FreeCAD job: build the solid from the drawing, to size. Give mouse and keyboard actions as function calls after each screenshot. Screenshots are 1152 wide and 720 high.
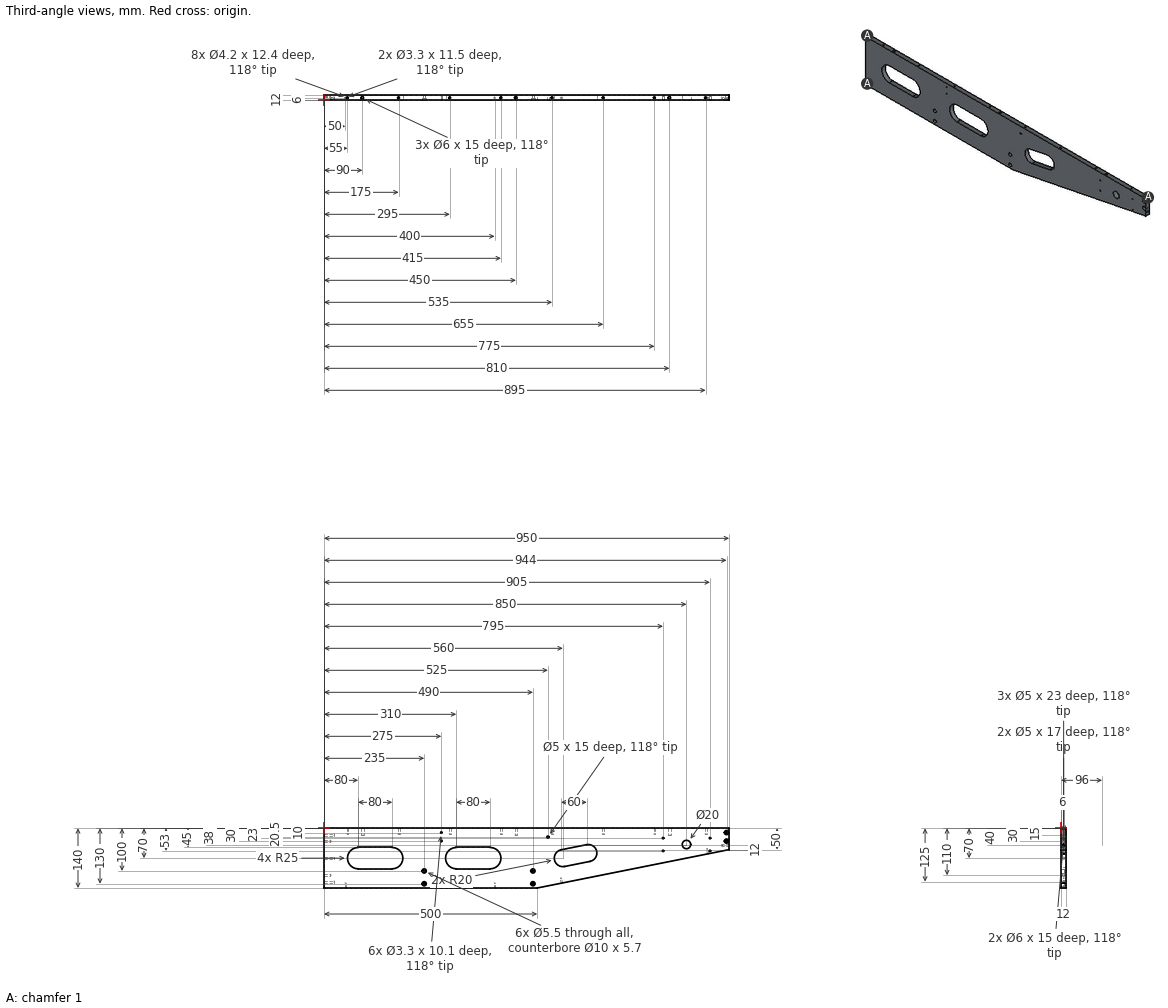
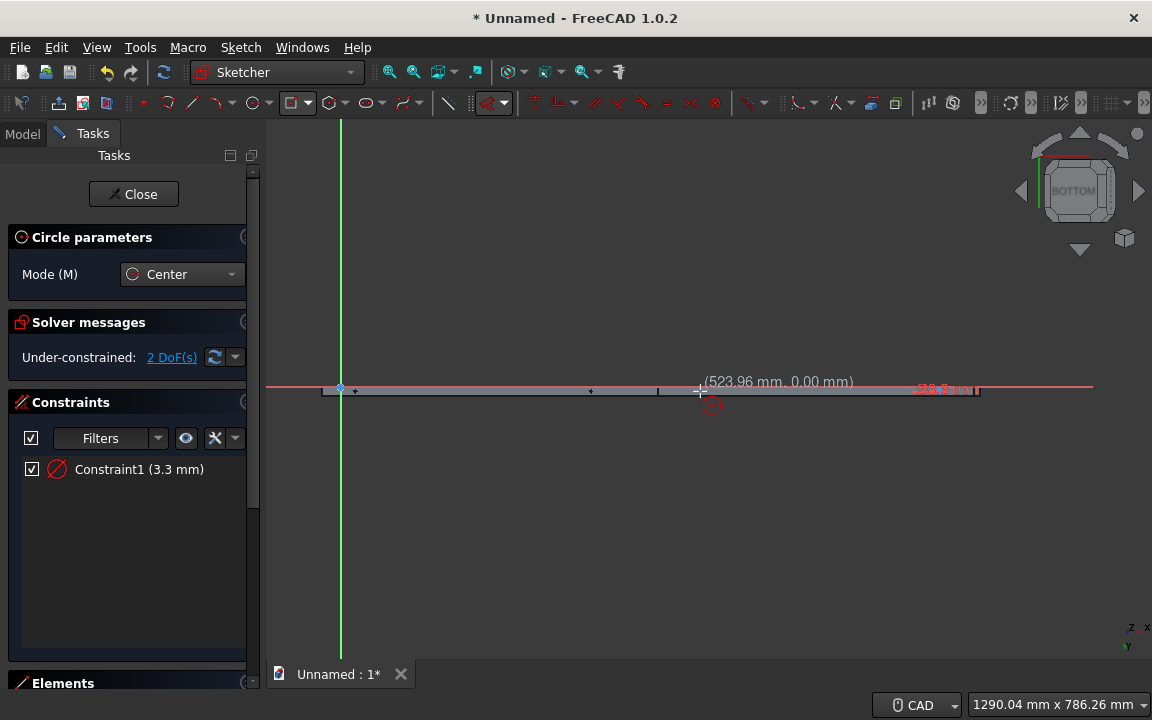
scroll(699, 391, up, 7)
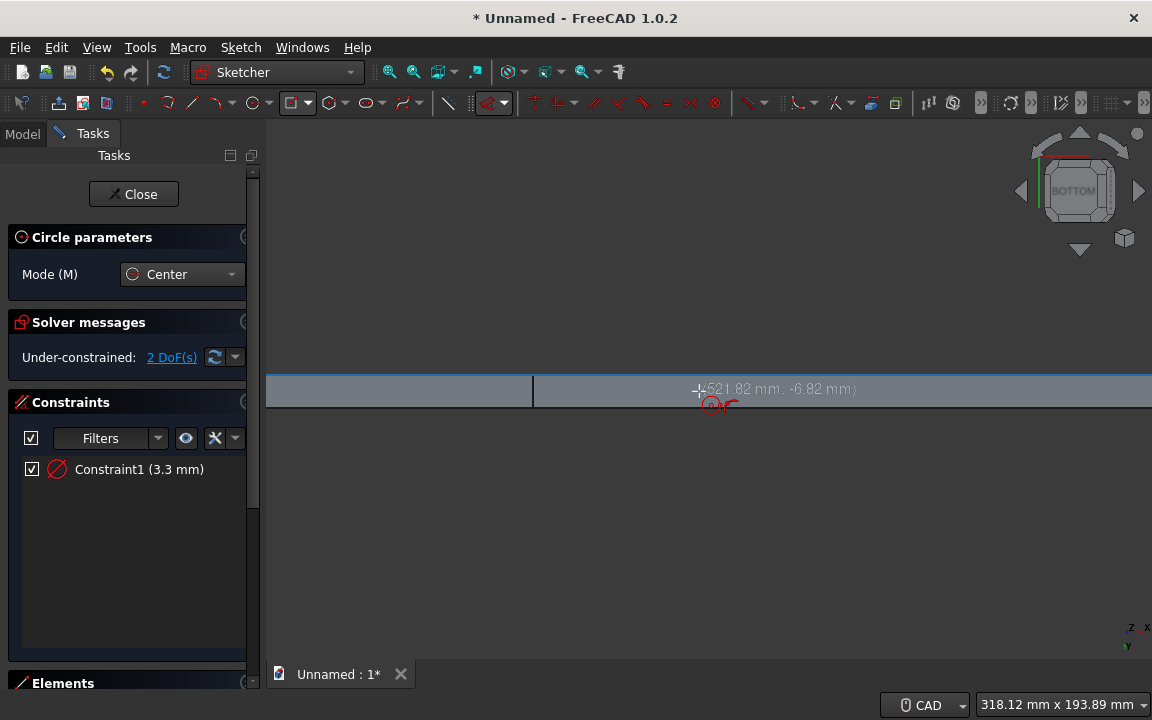
click(697, 391)
move(701, 394)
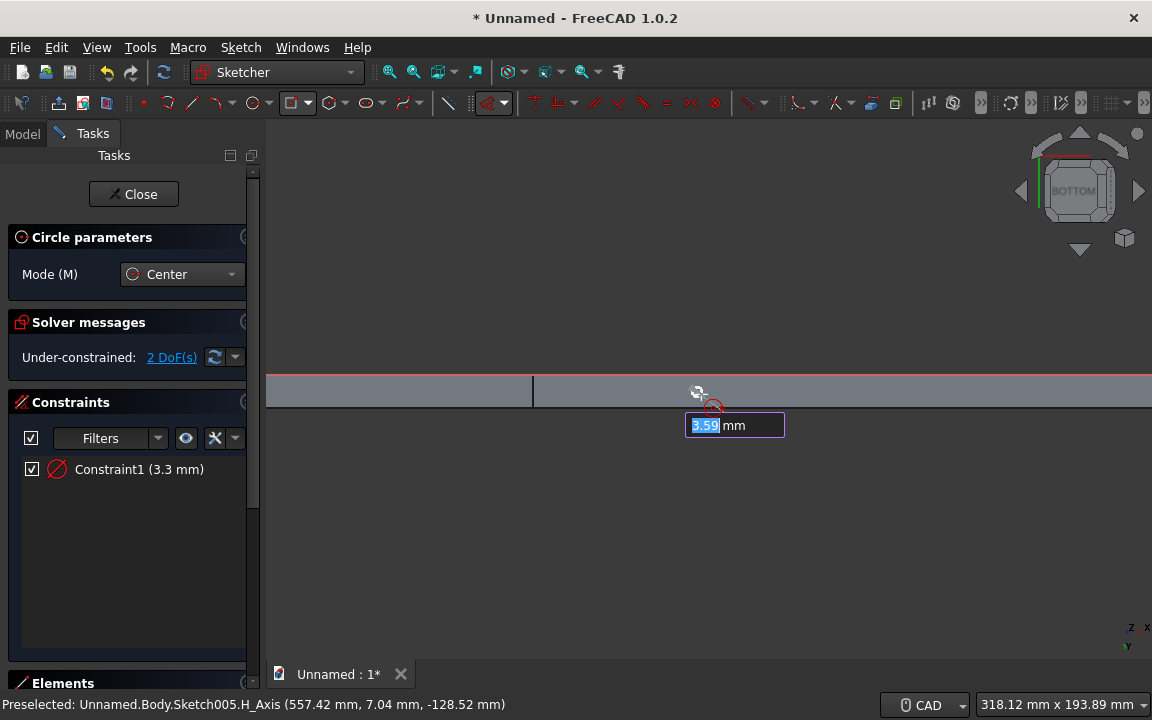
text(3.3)
key(Return)
key(Escape)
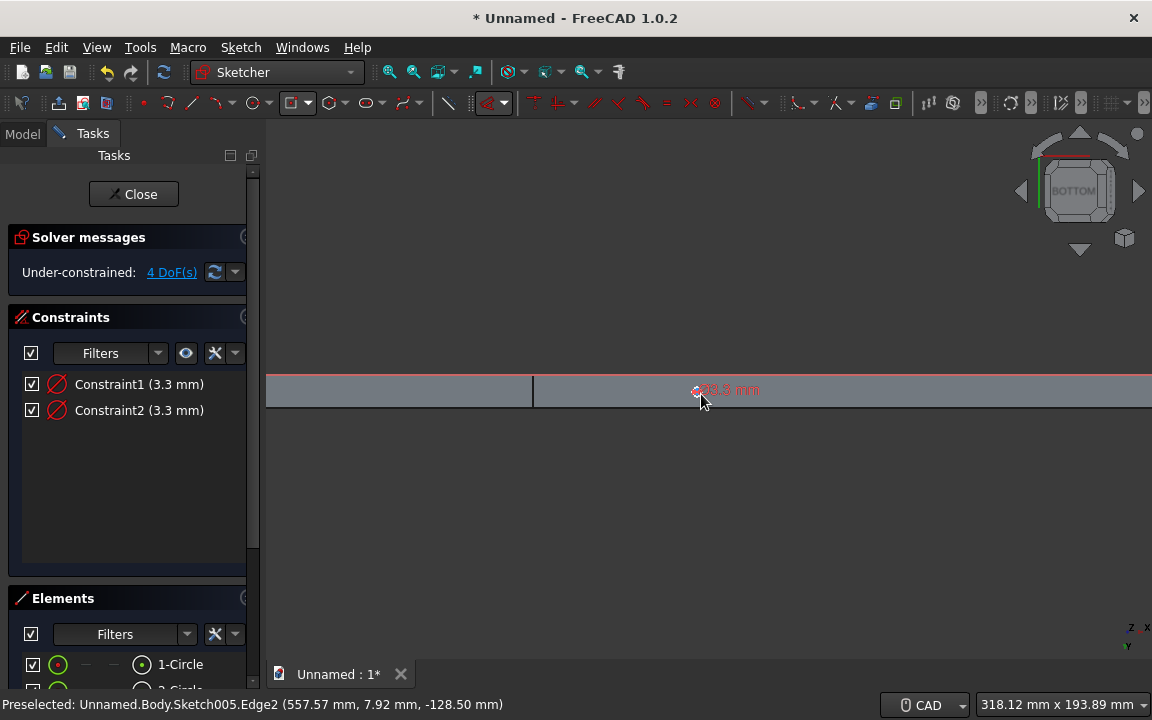
scroll(686, 390, down, 8)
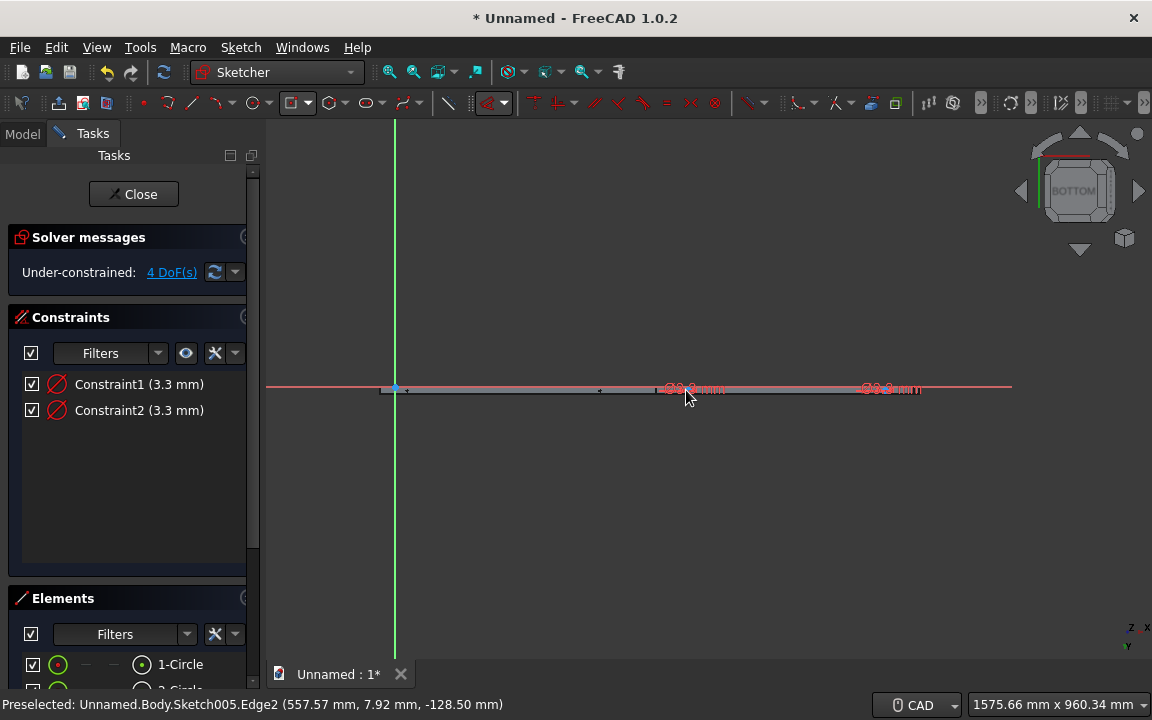
click(885, 391)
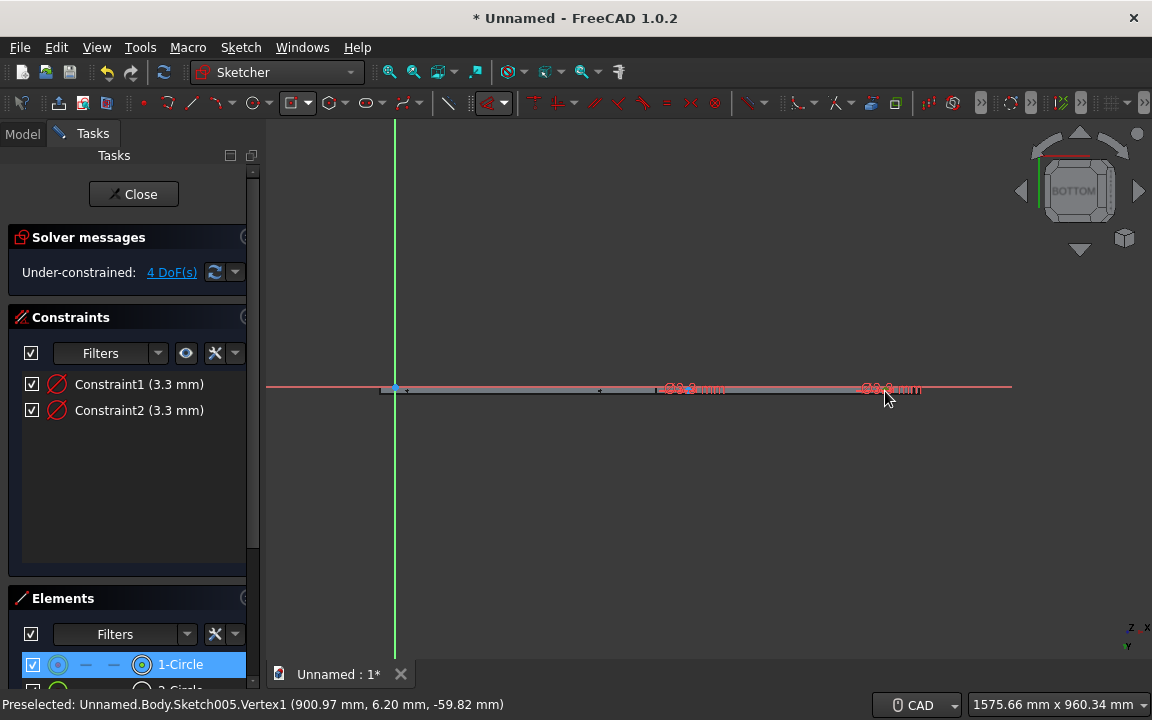
click(689, 391)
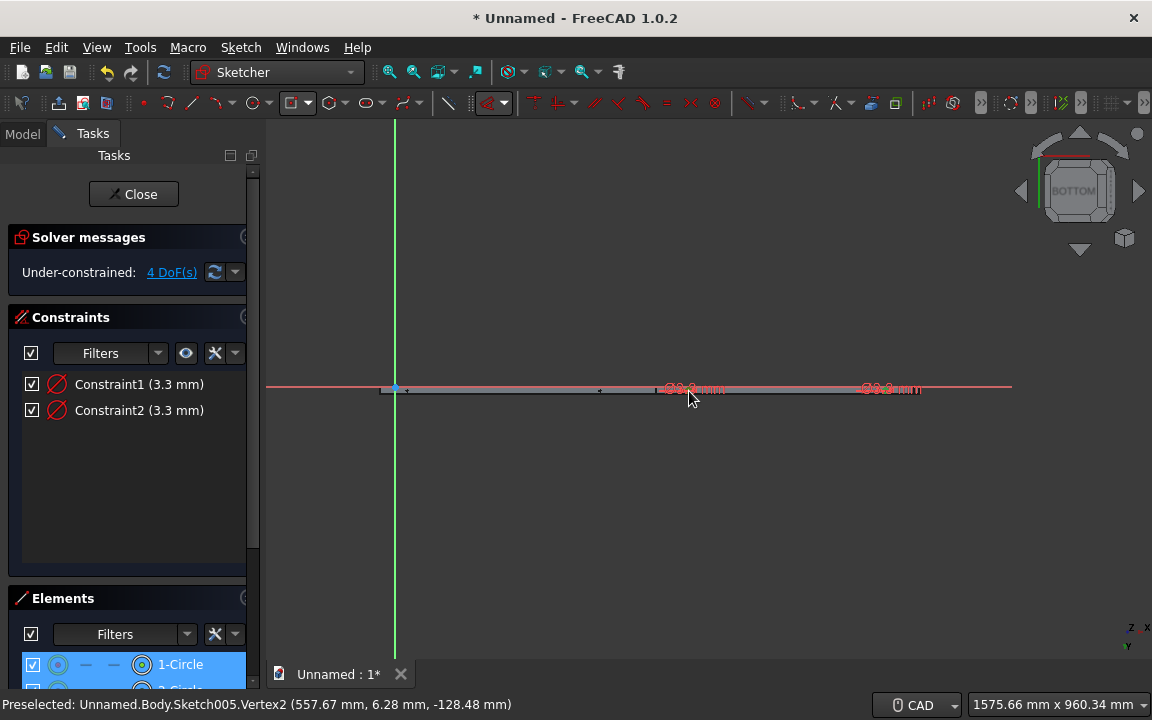
key(h)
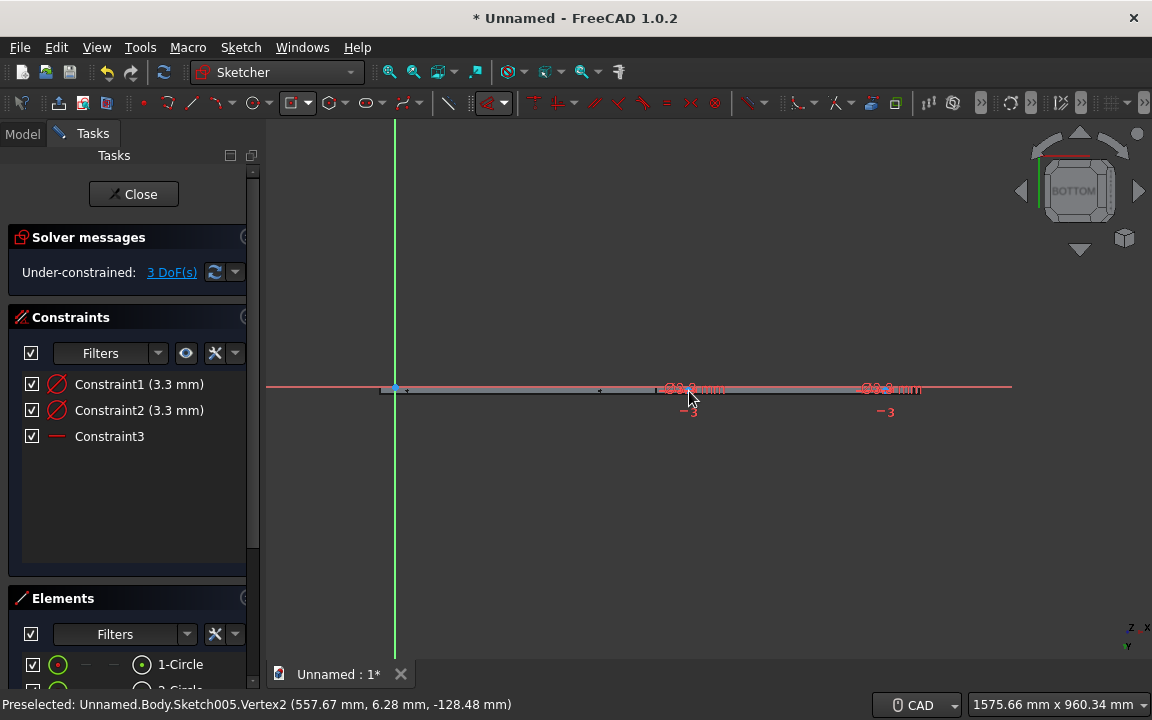
scroll(885, 391, up, 13)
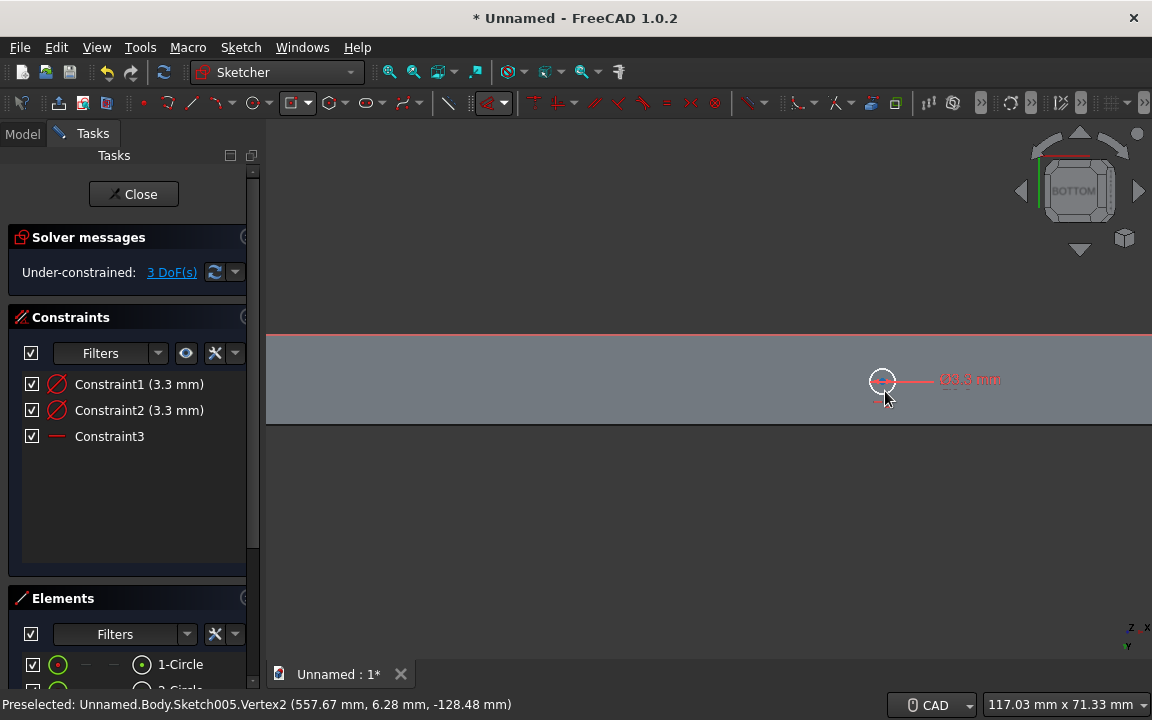
click(883, 382)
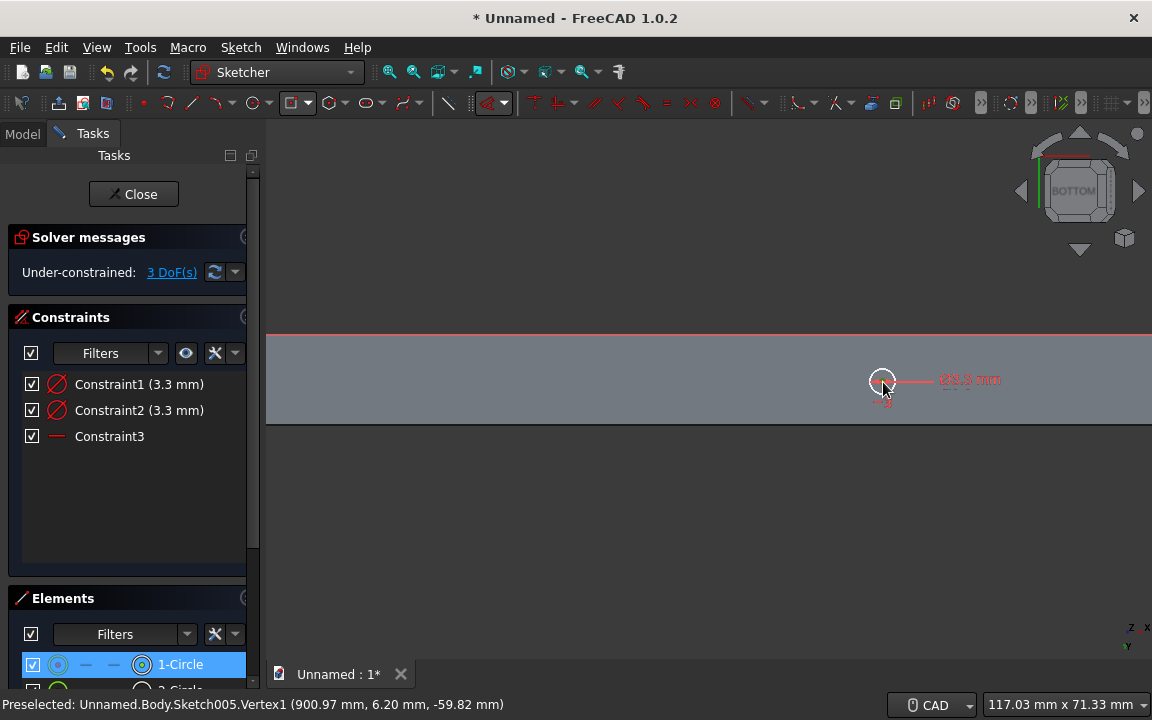
key(i)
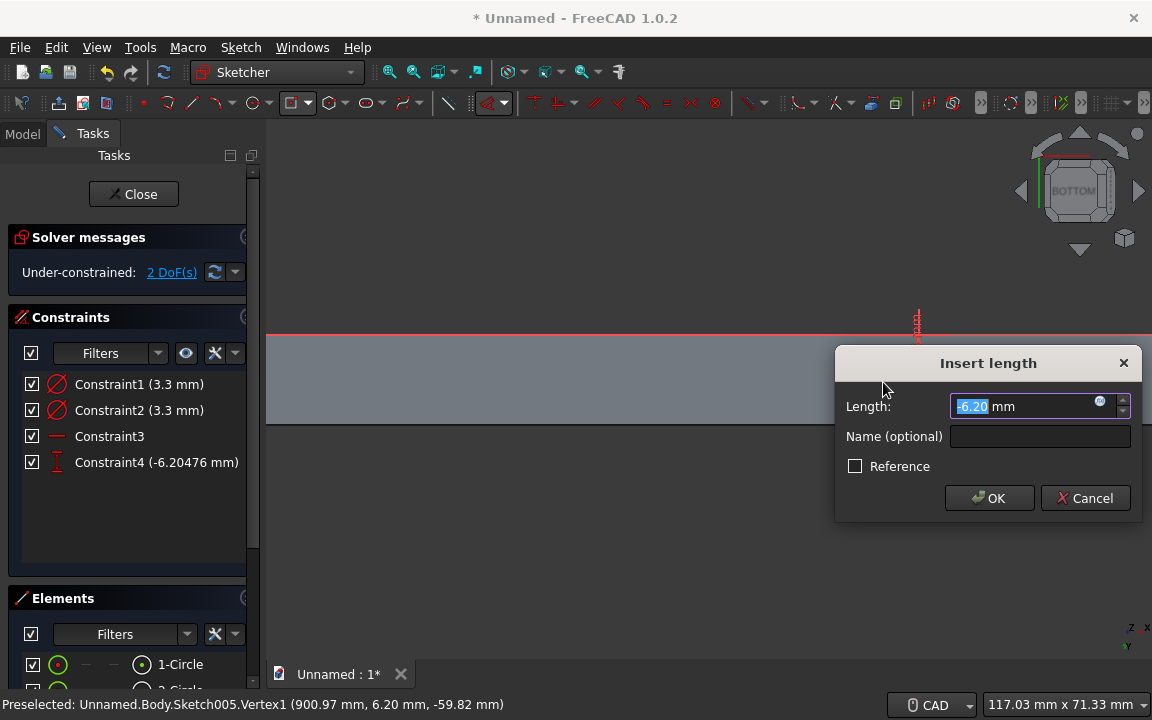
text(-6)
key(Return)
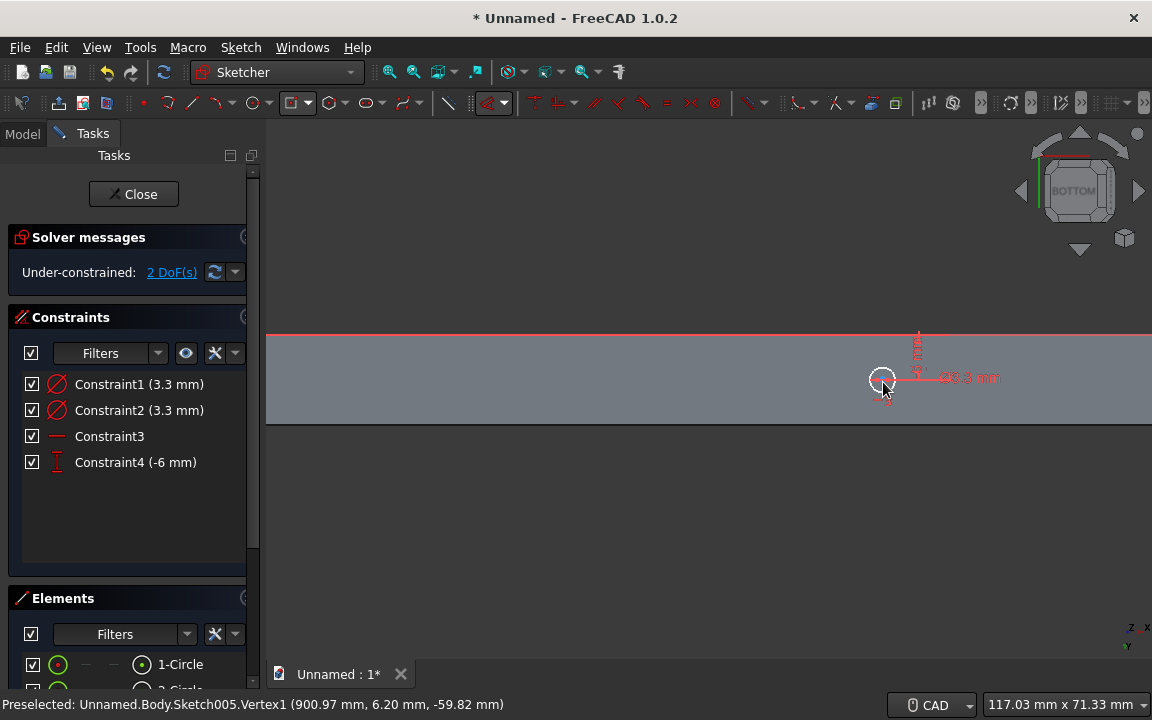
scroll(885, 391, down, 13)